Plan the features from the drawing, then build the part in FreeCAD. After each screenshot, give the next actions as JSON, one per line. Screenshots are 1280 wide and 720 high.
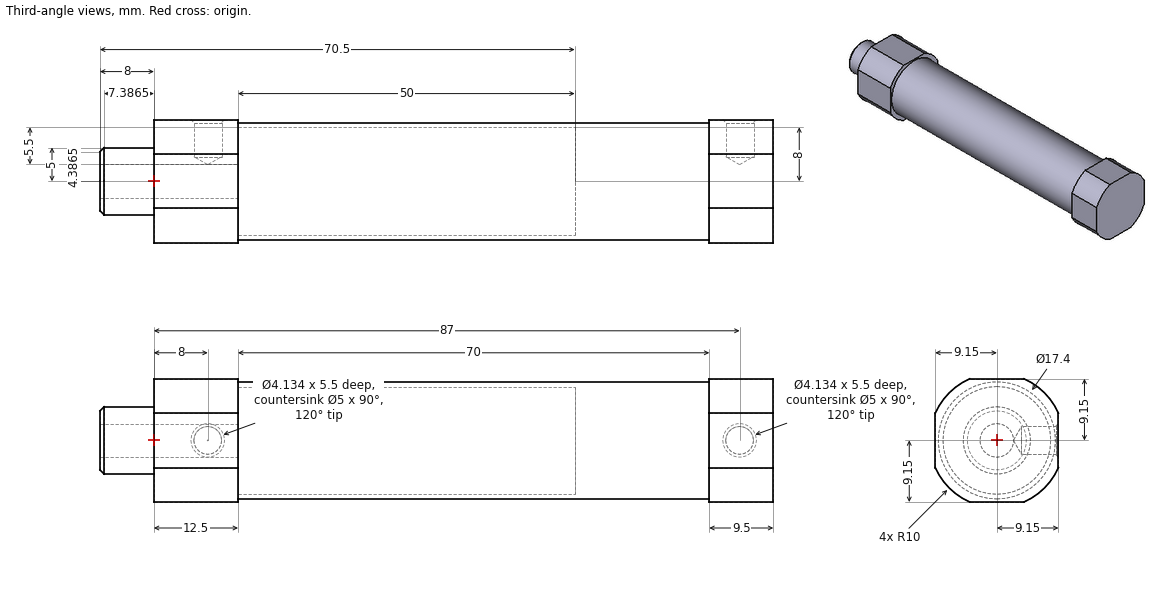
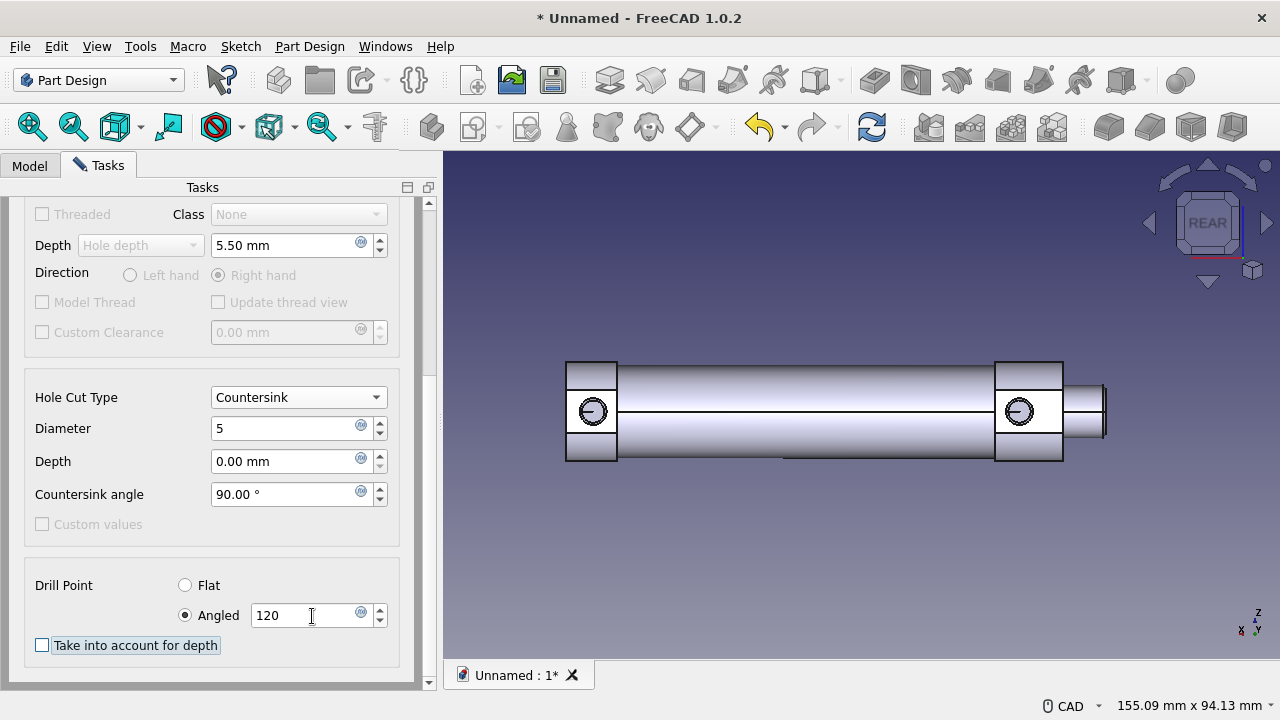
{"action": "scroll", "coordinate": [429, 444], "scroll_direction": "up", "scroll_amount": 6}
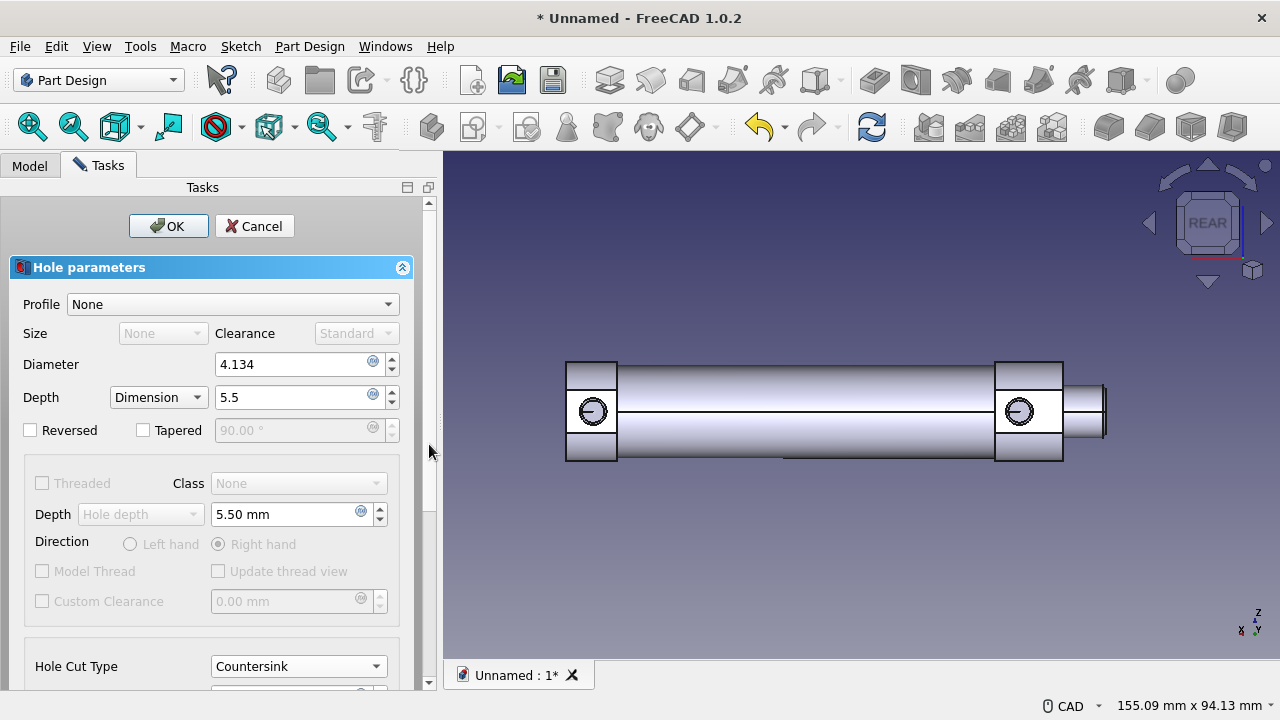
{"action": "left_click", "coordinate": [169, 226]}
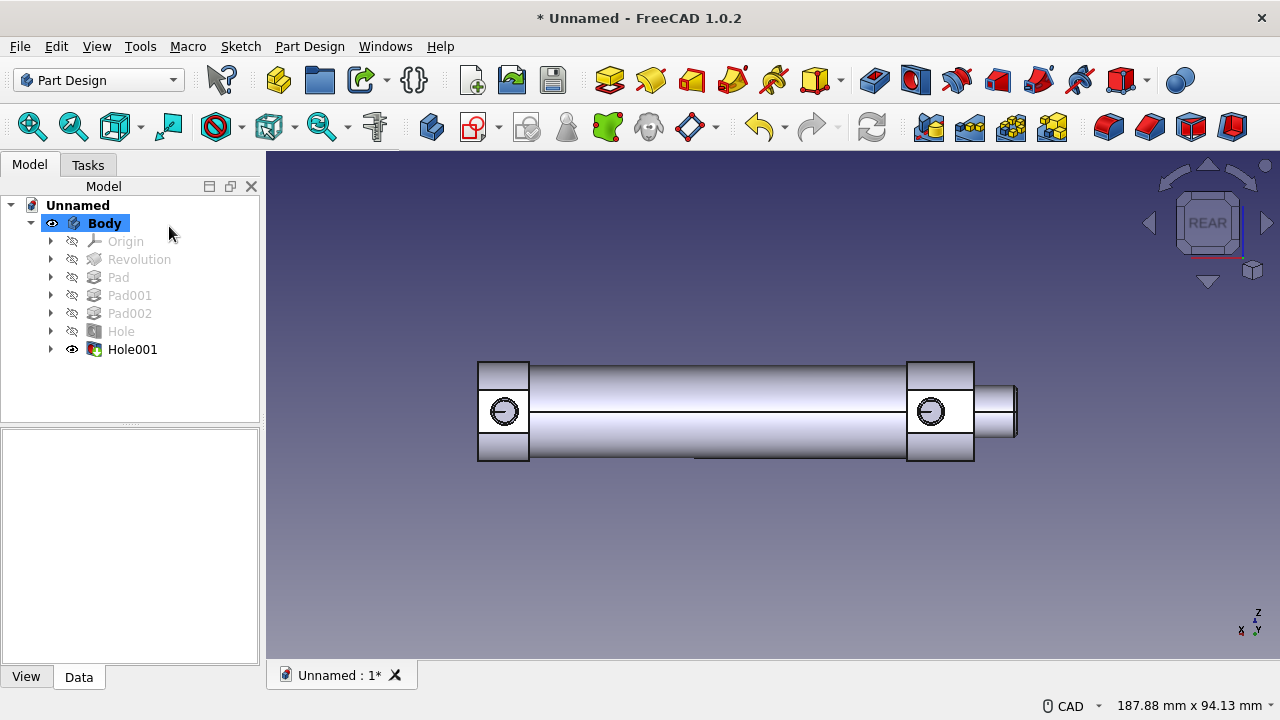
{"action": "left_click", "coordinate": [472, 128]}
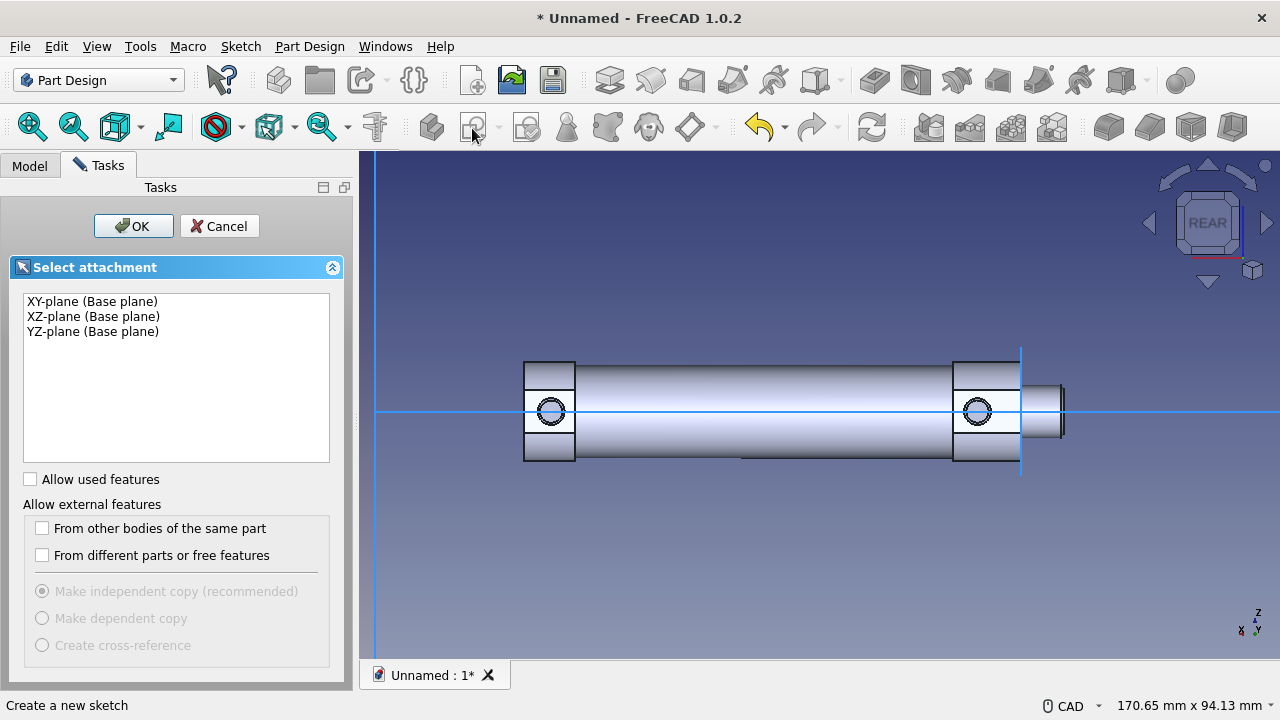
{"action": "left_click", "coordinate": [84, 302]}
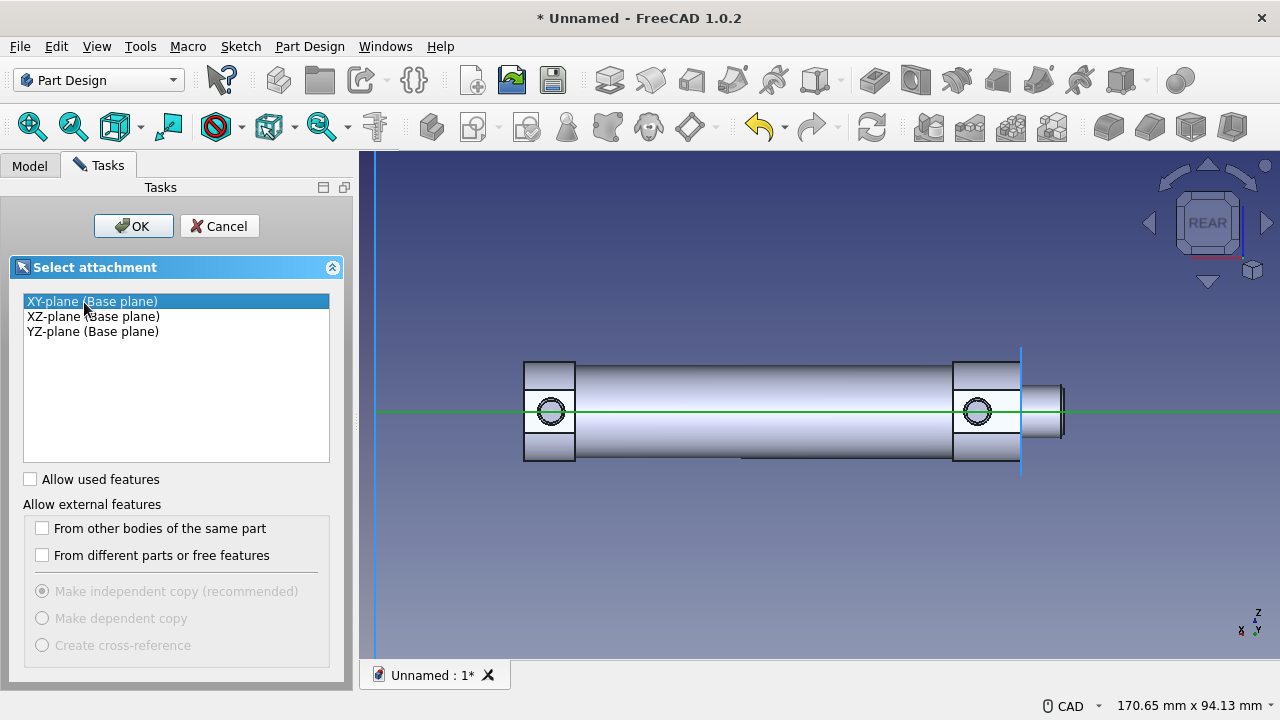
{"action": "left_click", "coordinate": [134, 226]}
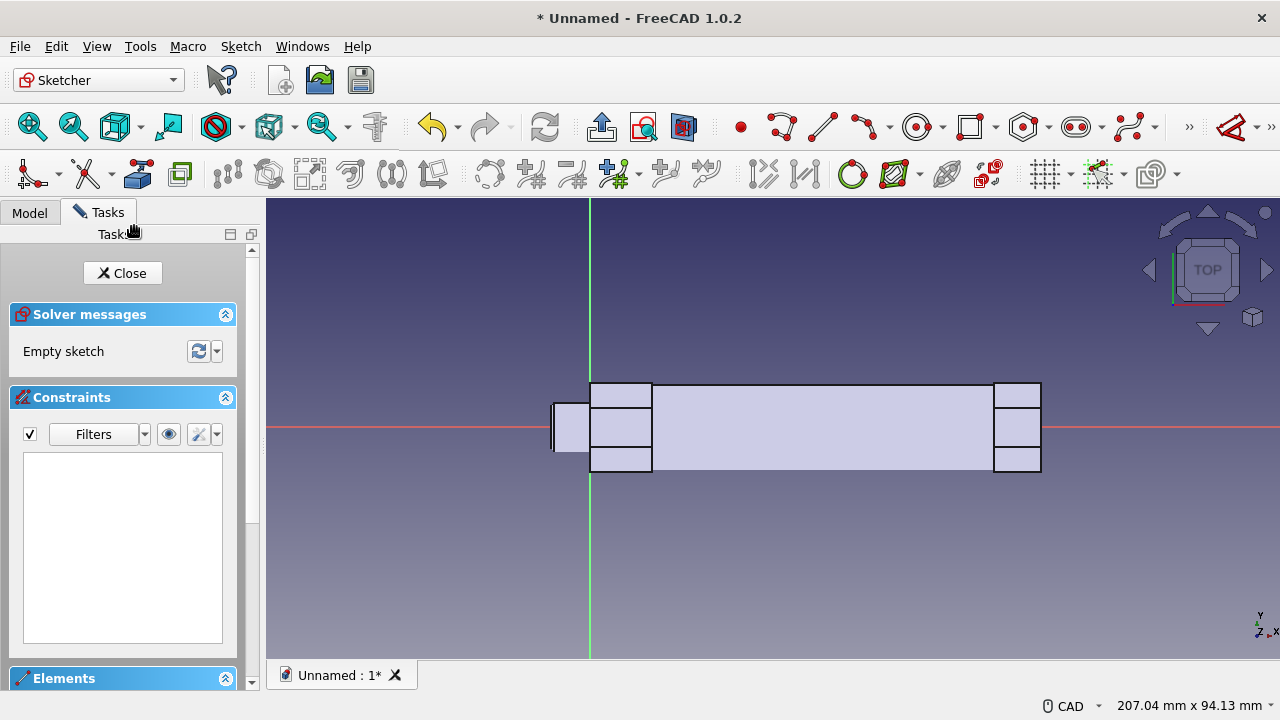
{"action": "left_click", "coordinate": [684, 128]}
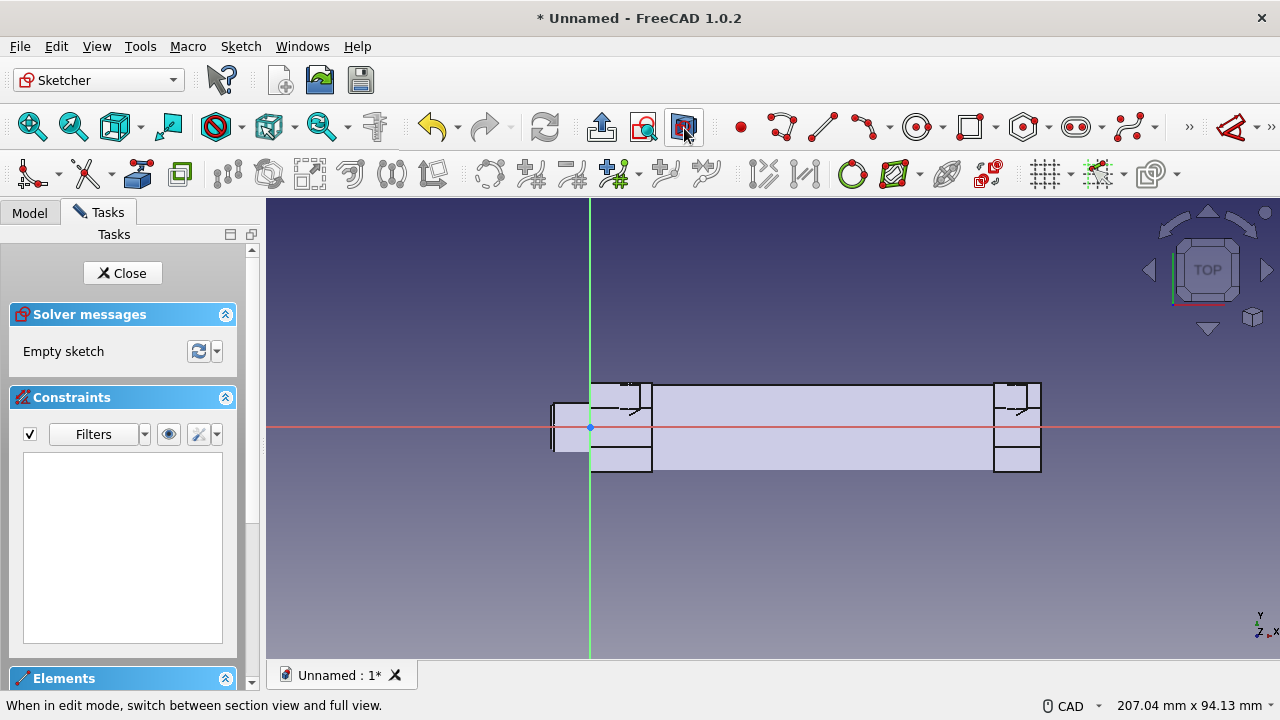
{"action": "scroll", "coordinate": [747, 383], "scroll_direction": "up", "scroll_amount": 3}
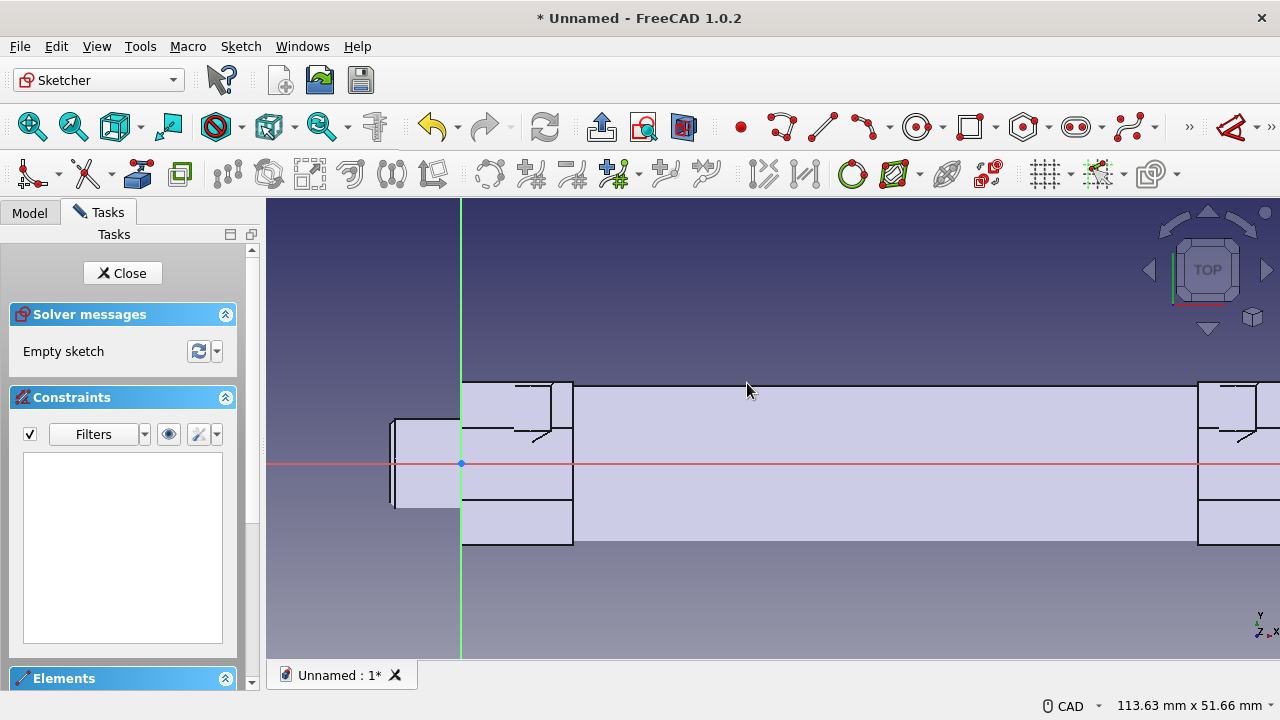
{"action": "left_click", "coordinate": [782, 128]}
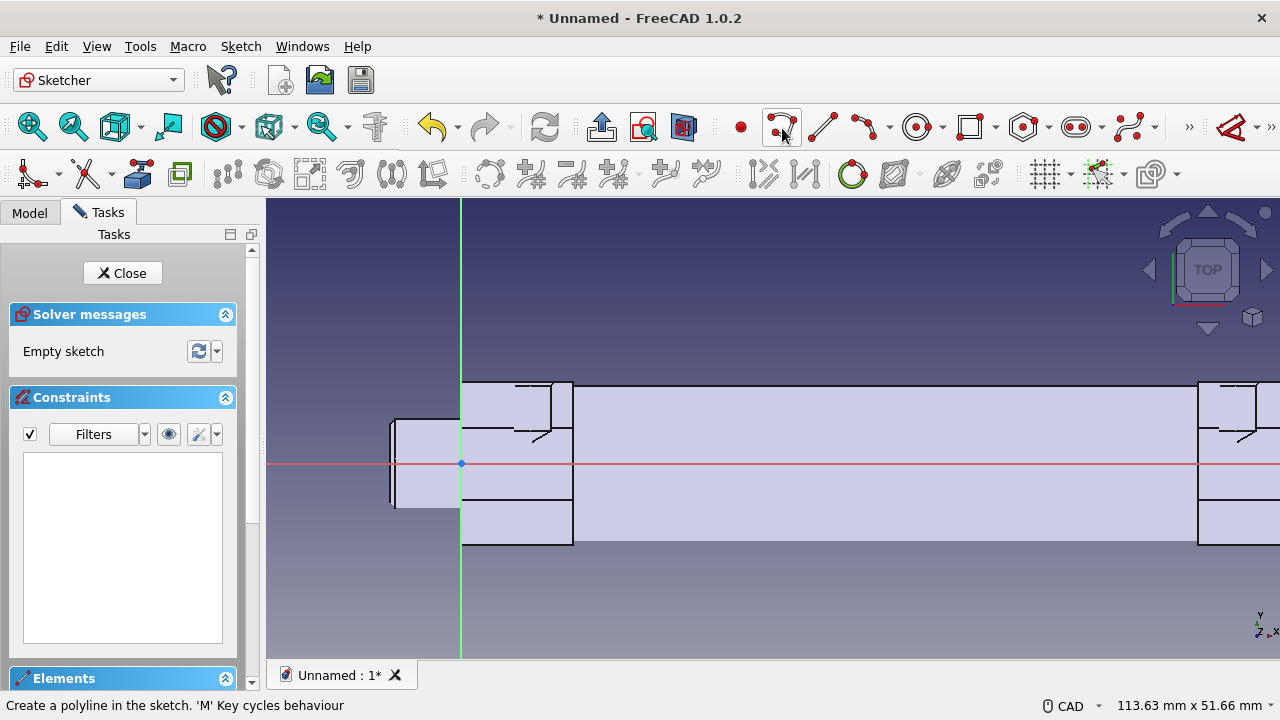
{"action": "left_click", "coordinate": [390, 464]}
{"action": "left_click", "coordinate": [1019, 455]}
{"action": "left_click", "coordinate": [1019, 392]}
{"action": "left_click", "coordinate": [573, 392]}
{"action": "left_click", "coordinate": [573, 441]}
{"action": "left_click", "coordinate": [390, 441]}
{"action": "left_click", "coordinate": [390, 464]}
{"action": "key", "text": "Escape"}
{"action": "key", "text": "Escape"}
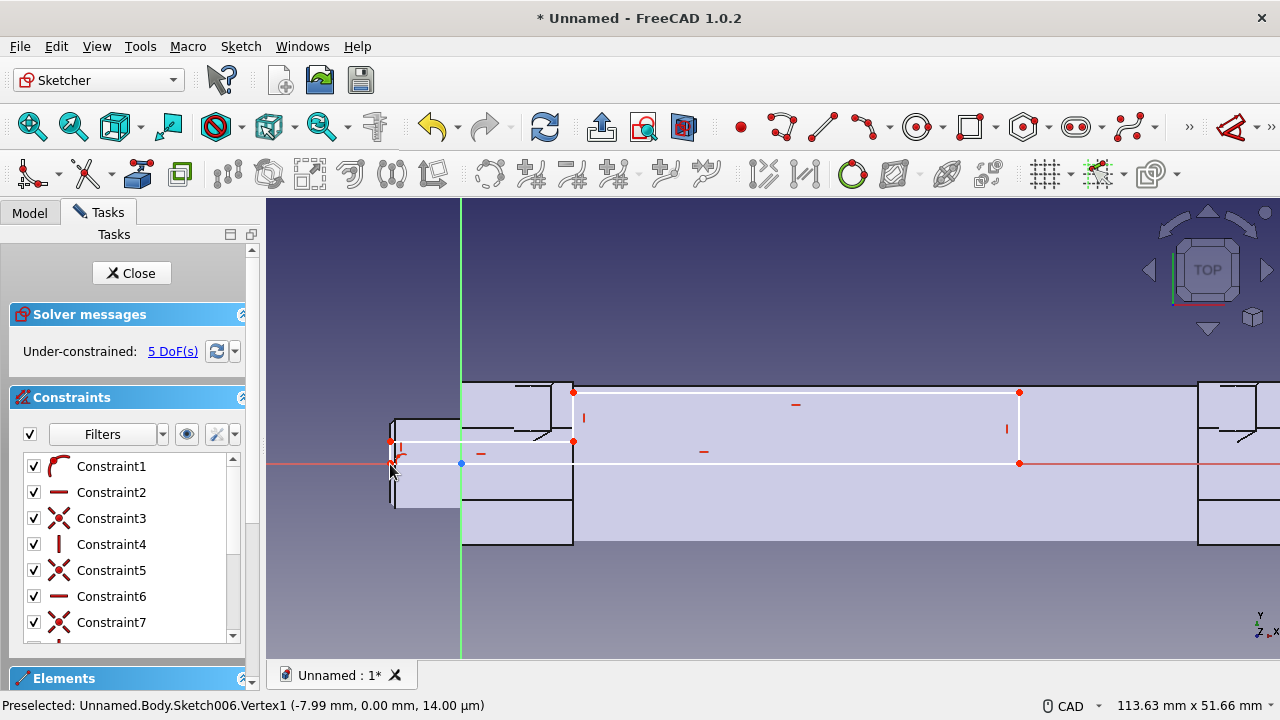
{"action": "key", "text": "d"}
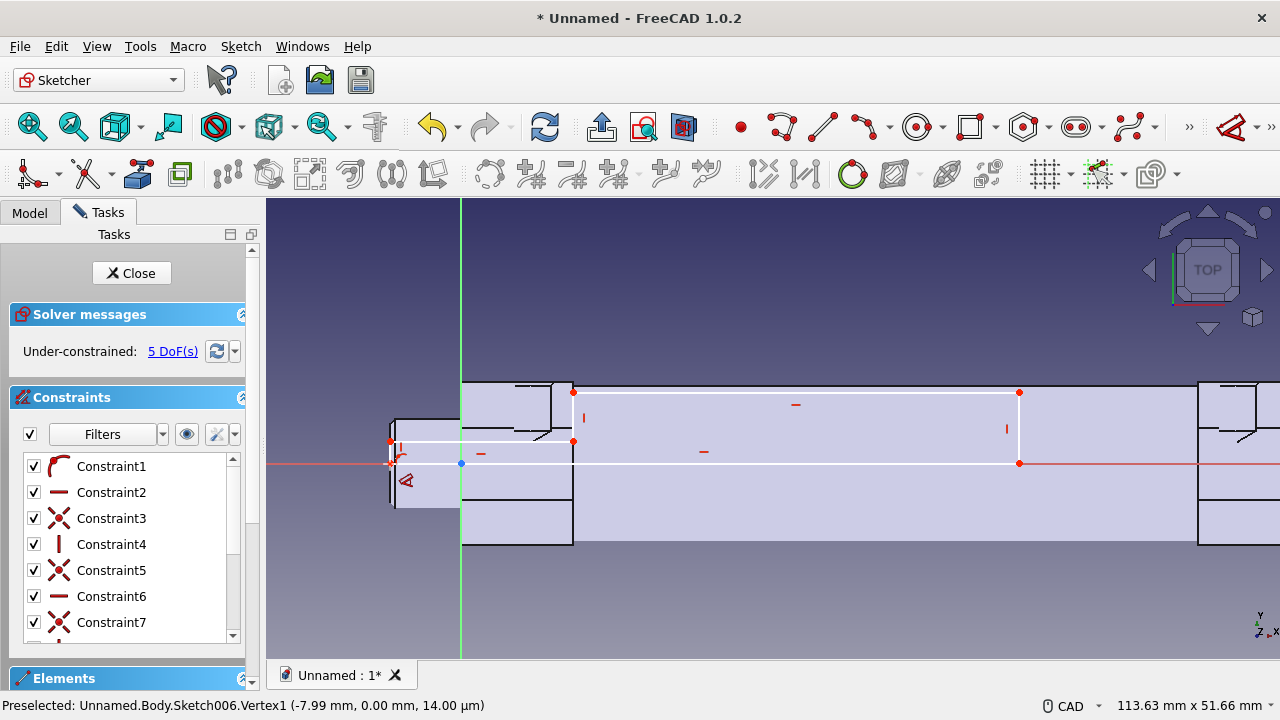
{"action": "left_click", "coordinate": [1019, 442]}
{"action": "left_click", "coordinate": [1053, 428]}